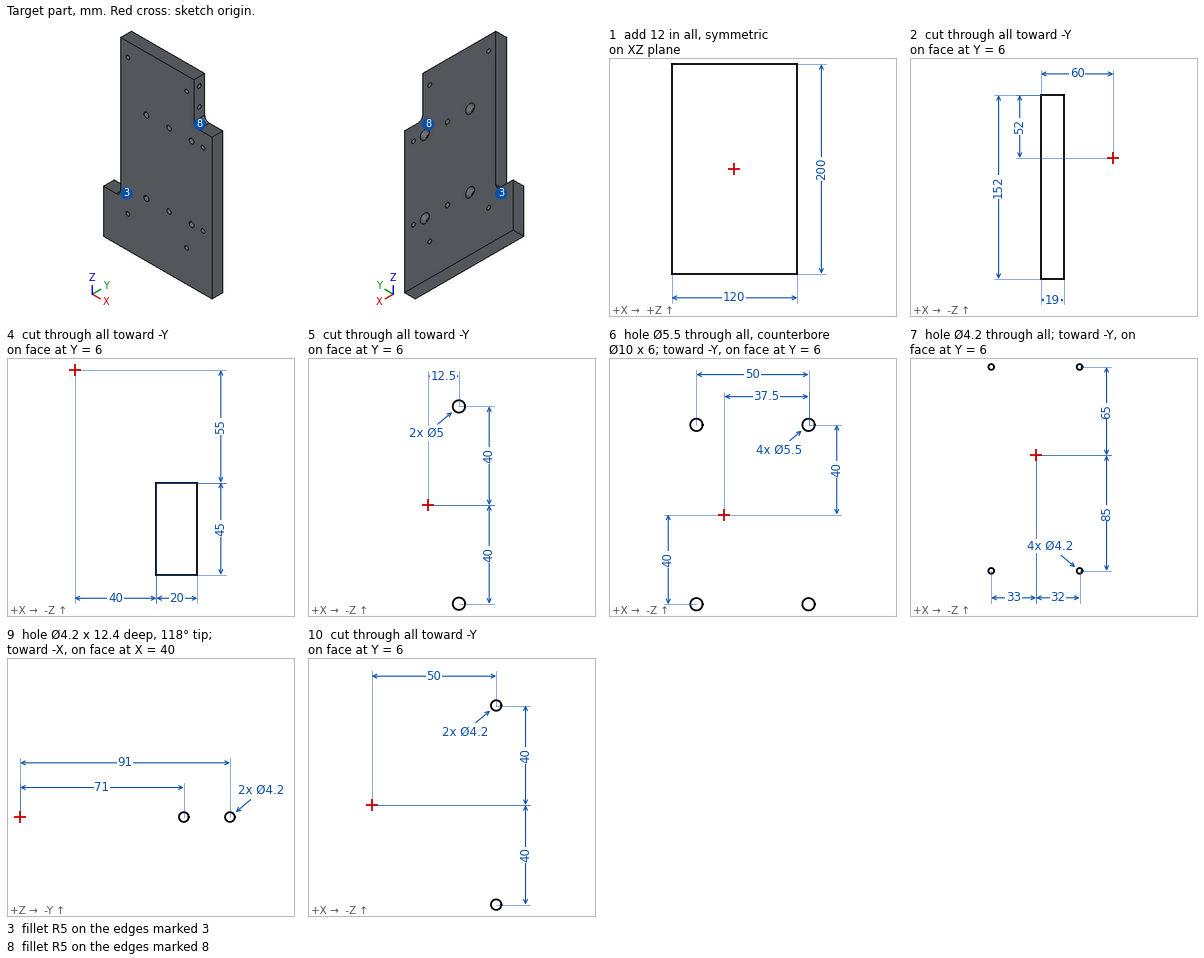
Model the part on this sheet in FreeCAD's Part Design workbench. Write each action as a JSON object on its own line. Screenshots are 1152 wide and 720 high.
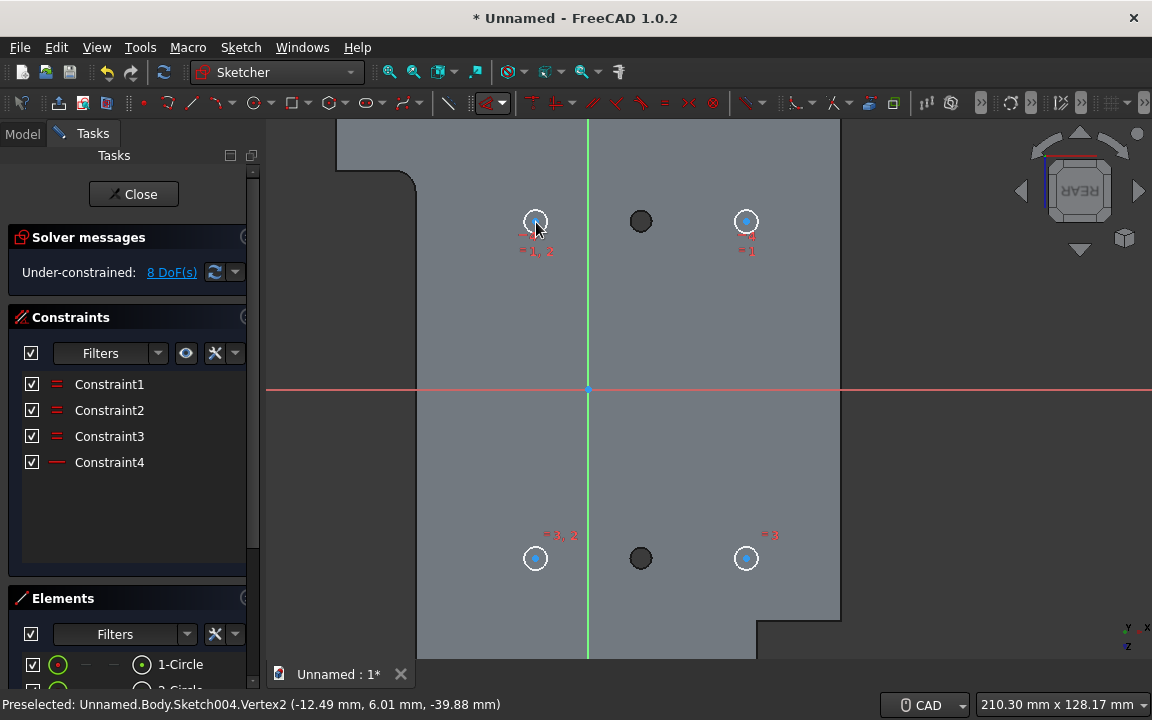
{"action": "left_click", "coordinate": [536, 222]}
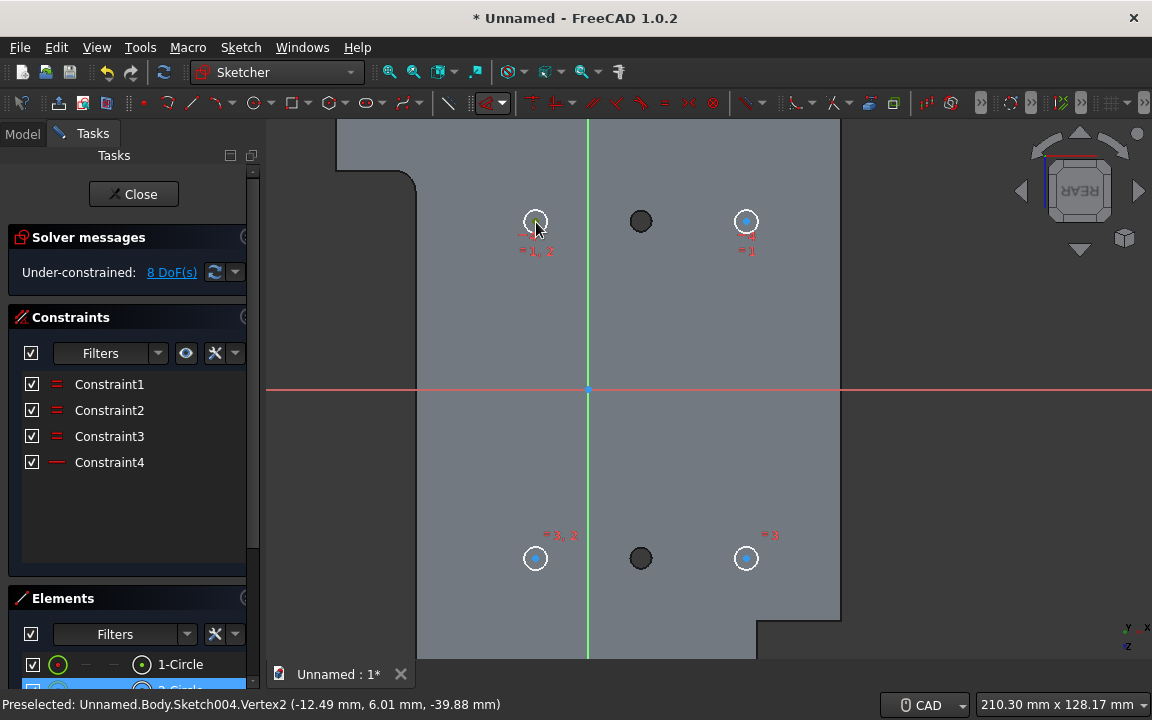
{"action": "left_click", "coordinate": [536, 559]}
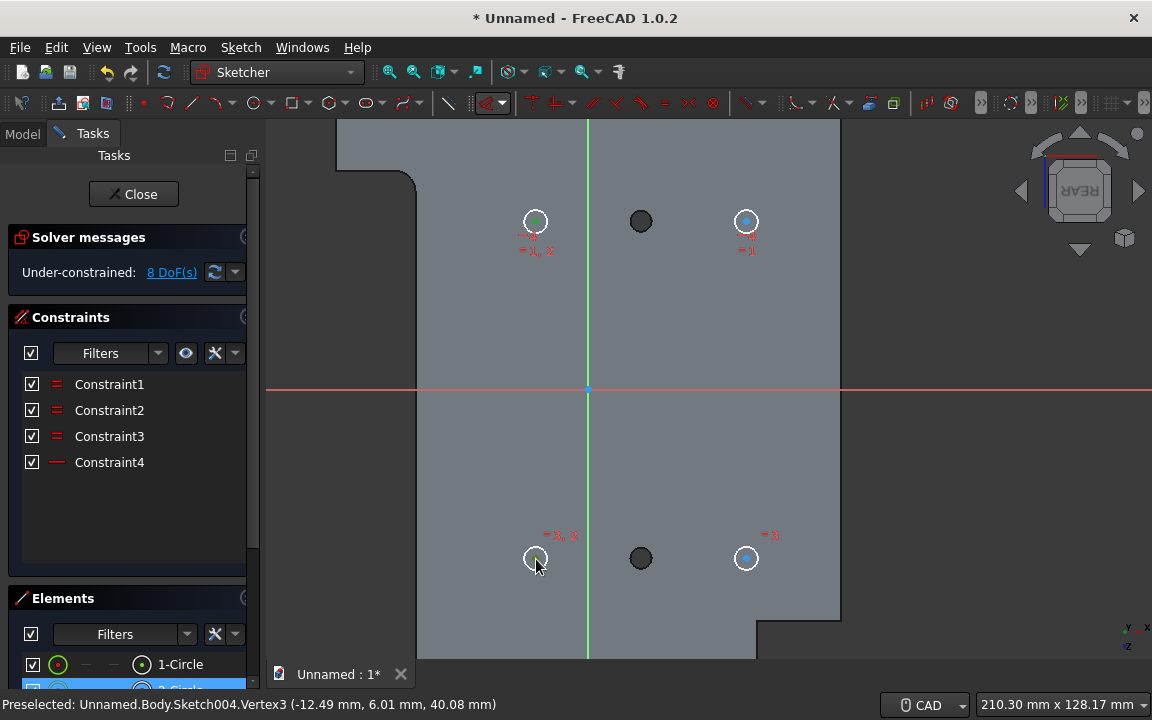
{"action": "key", "text": "v"}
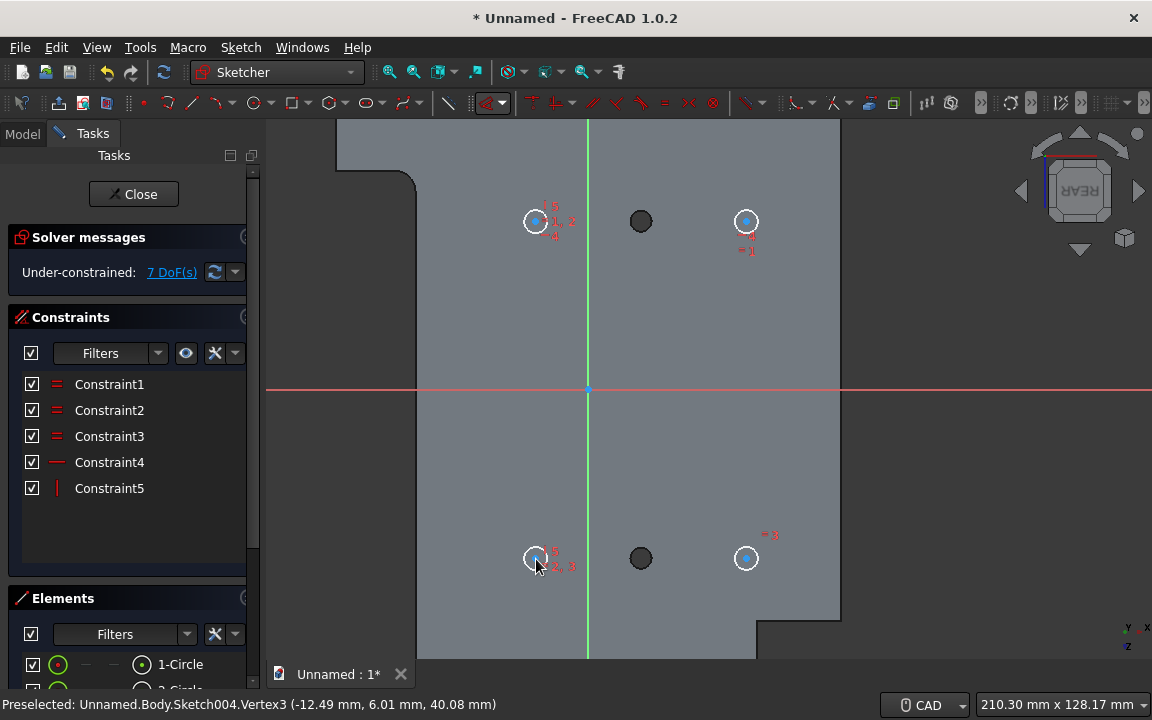
{"action": "left_click", "coordinate": [746, 222]}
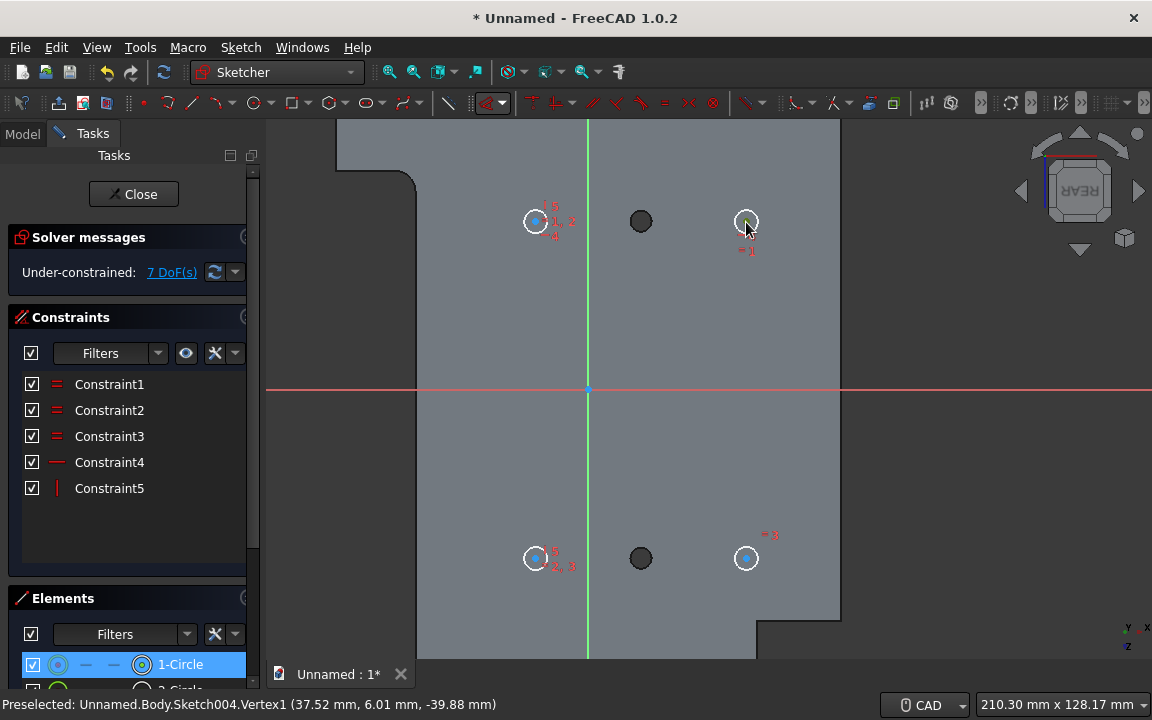
{"action": "left_click", "coordinate": [746, 558]}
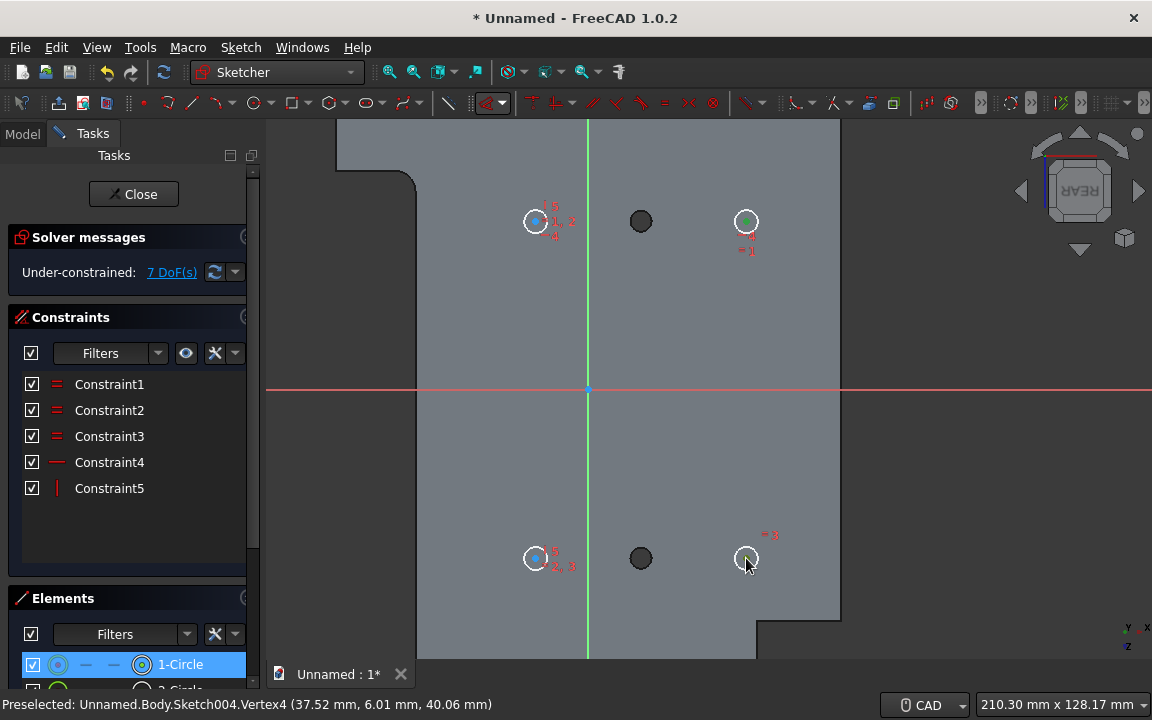
{"action": "left_click", "coordinate": [574, 104]}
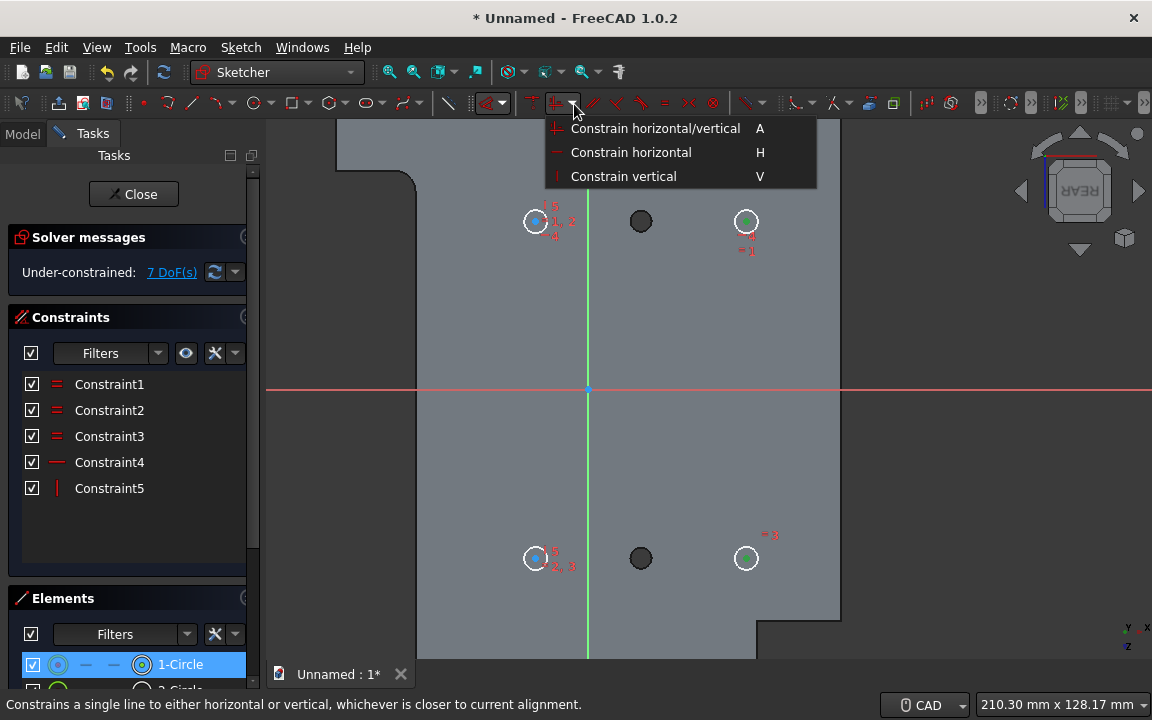
{"action": "left_click", "coordinate": [681, 176]}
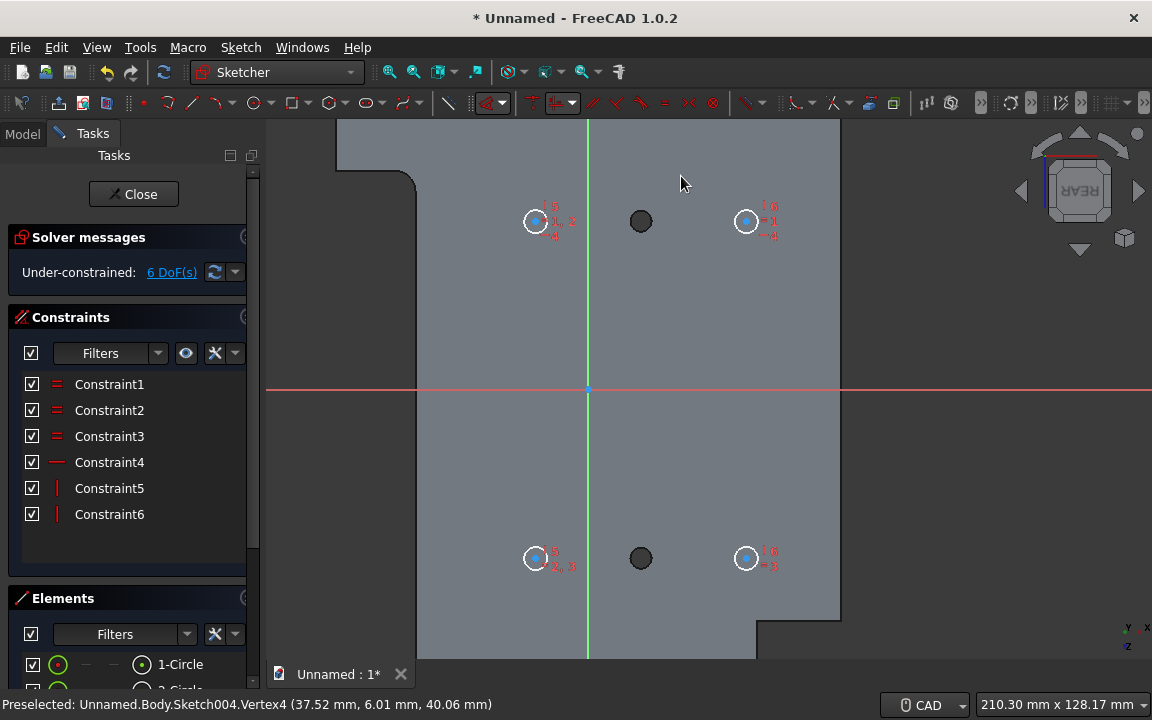
{"action": "left_click", "coordinate": [536, 559]}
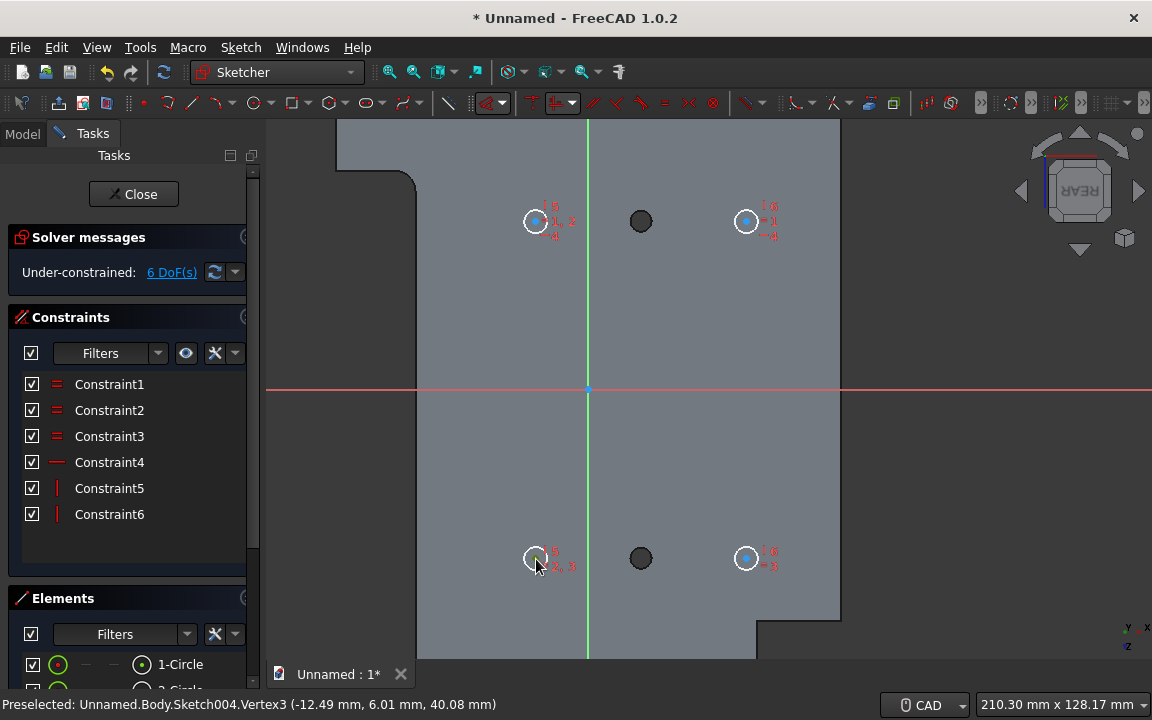
{"action": "left_click", "coordinate": [746, 558]}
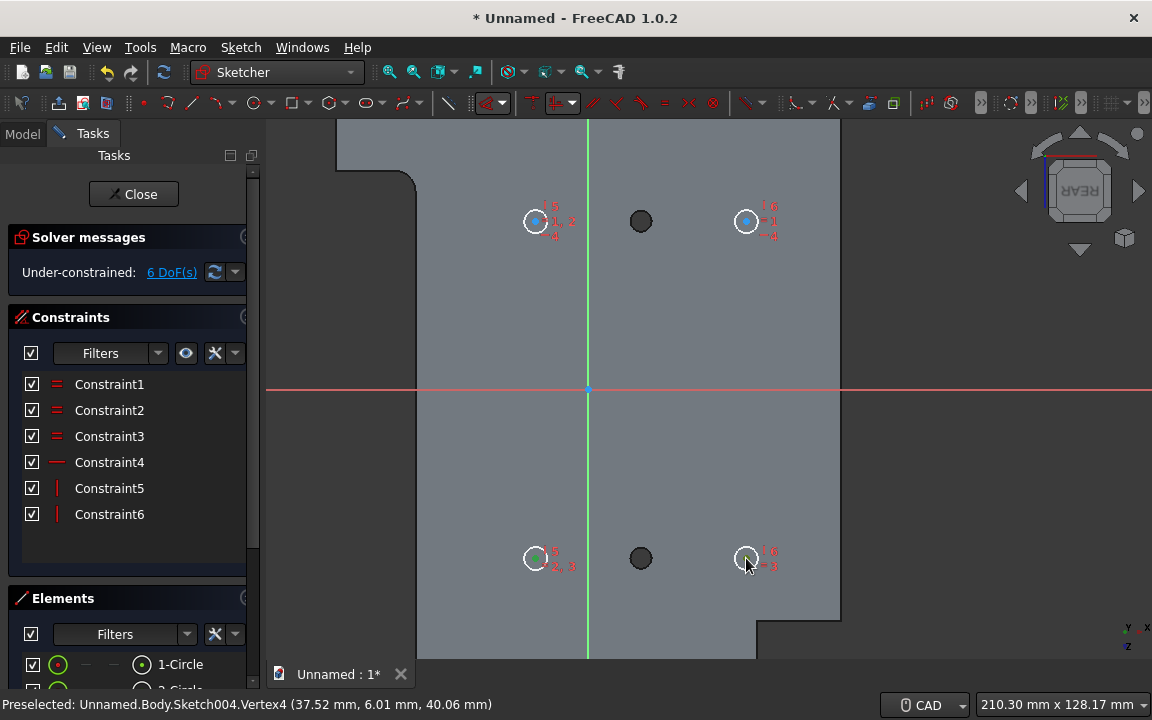
{"action": "key", "text": "h"}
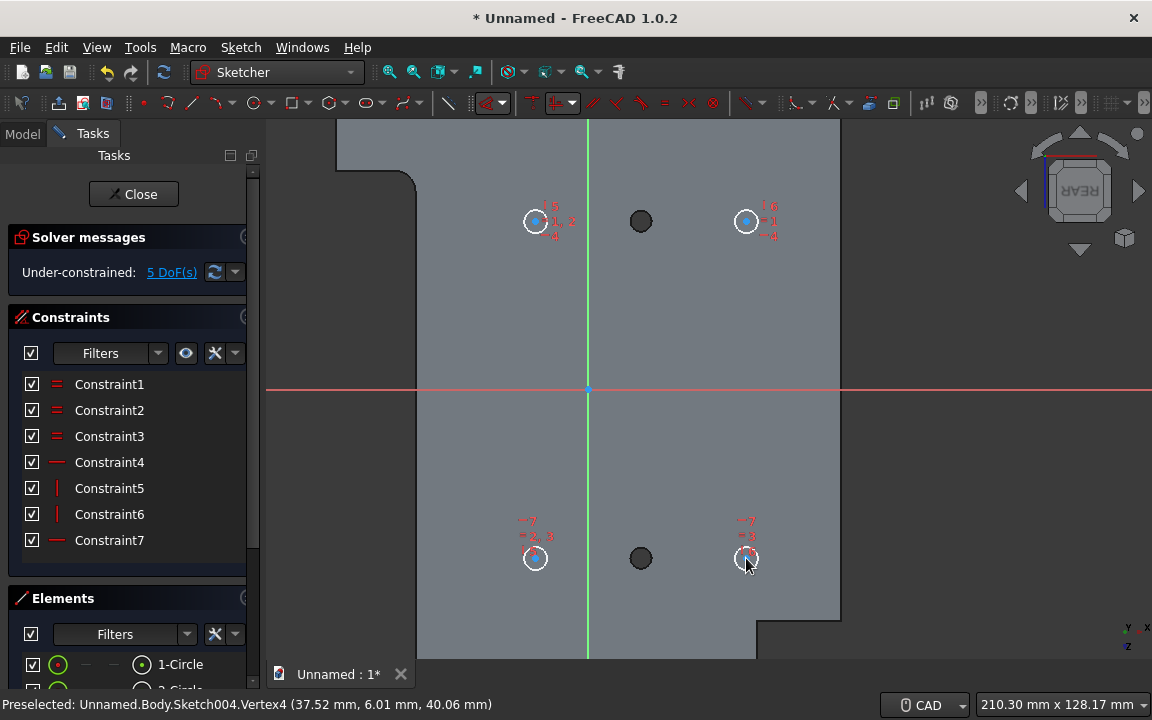
{"action": "scroll", "coordinate": [754, 214], "scroll_direction": "up", "scroll_amount": 3}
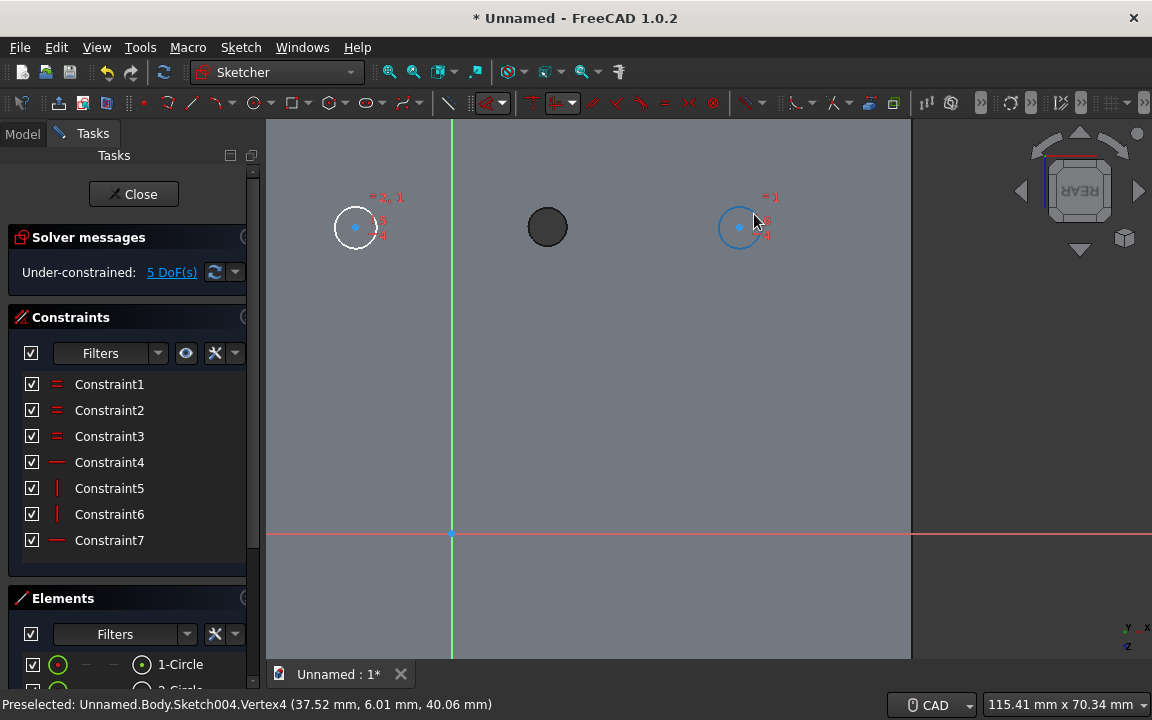
{"action": "left_click", "coordinate": [725, 213]}